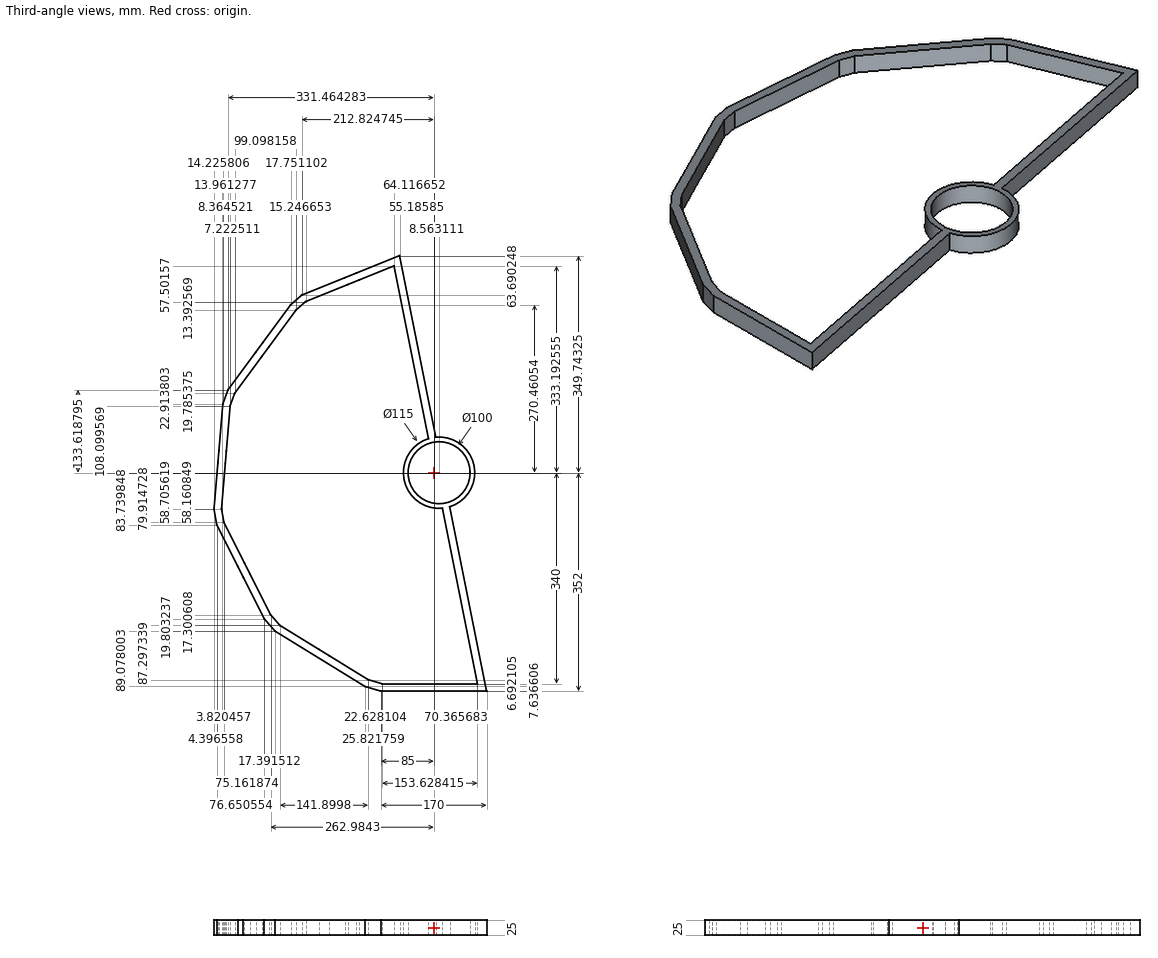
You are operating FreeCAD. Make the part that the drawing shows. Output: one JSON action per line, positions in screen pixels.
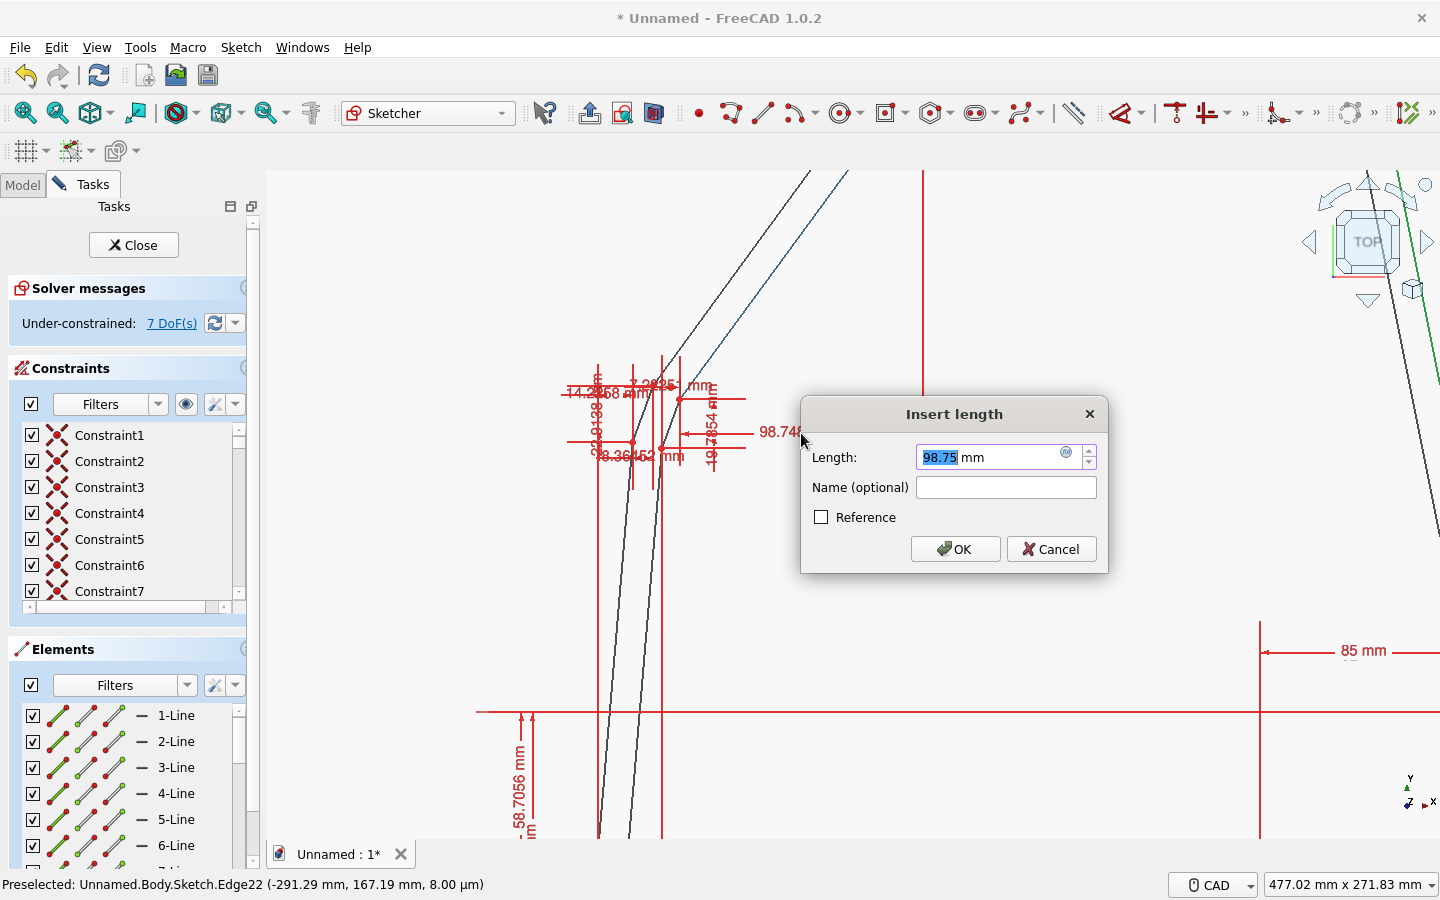
{"action": "type", "text": "99.098158"}
{"action": "key", "text": "Return"}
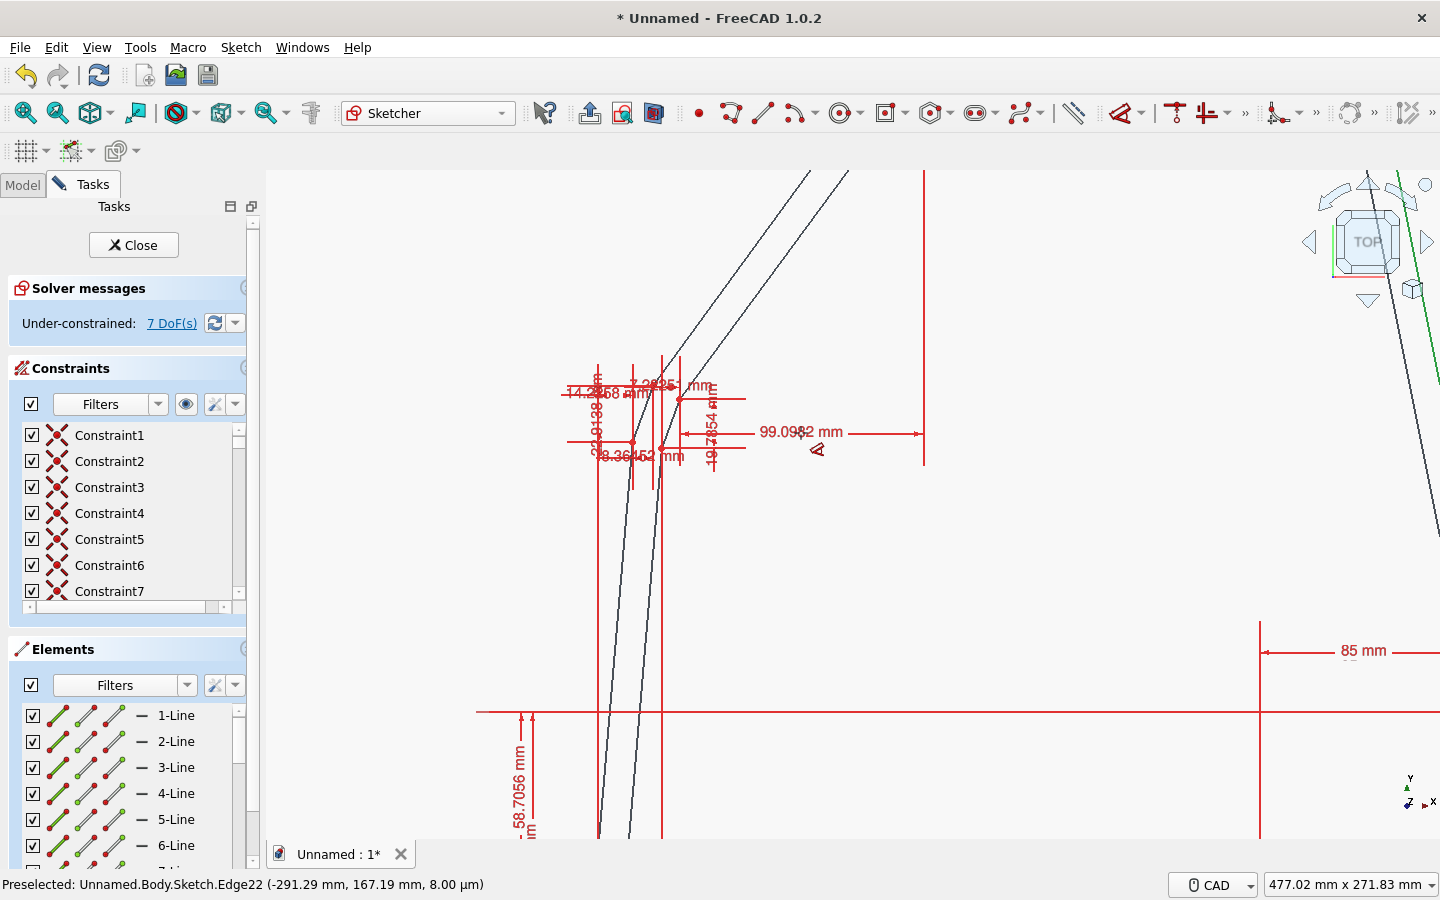
{"action": "scroll", "coordinate": [669, 436], "scroll_direction": "down", "scroll_amount": 7}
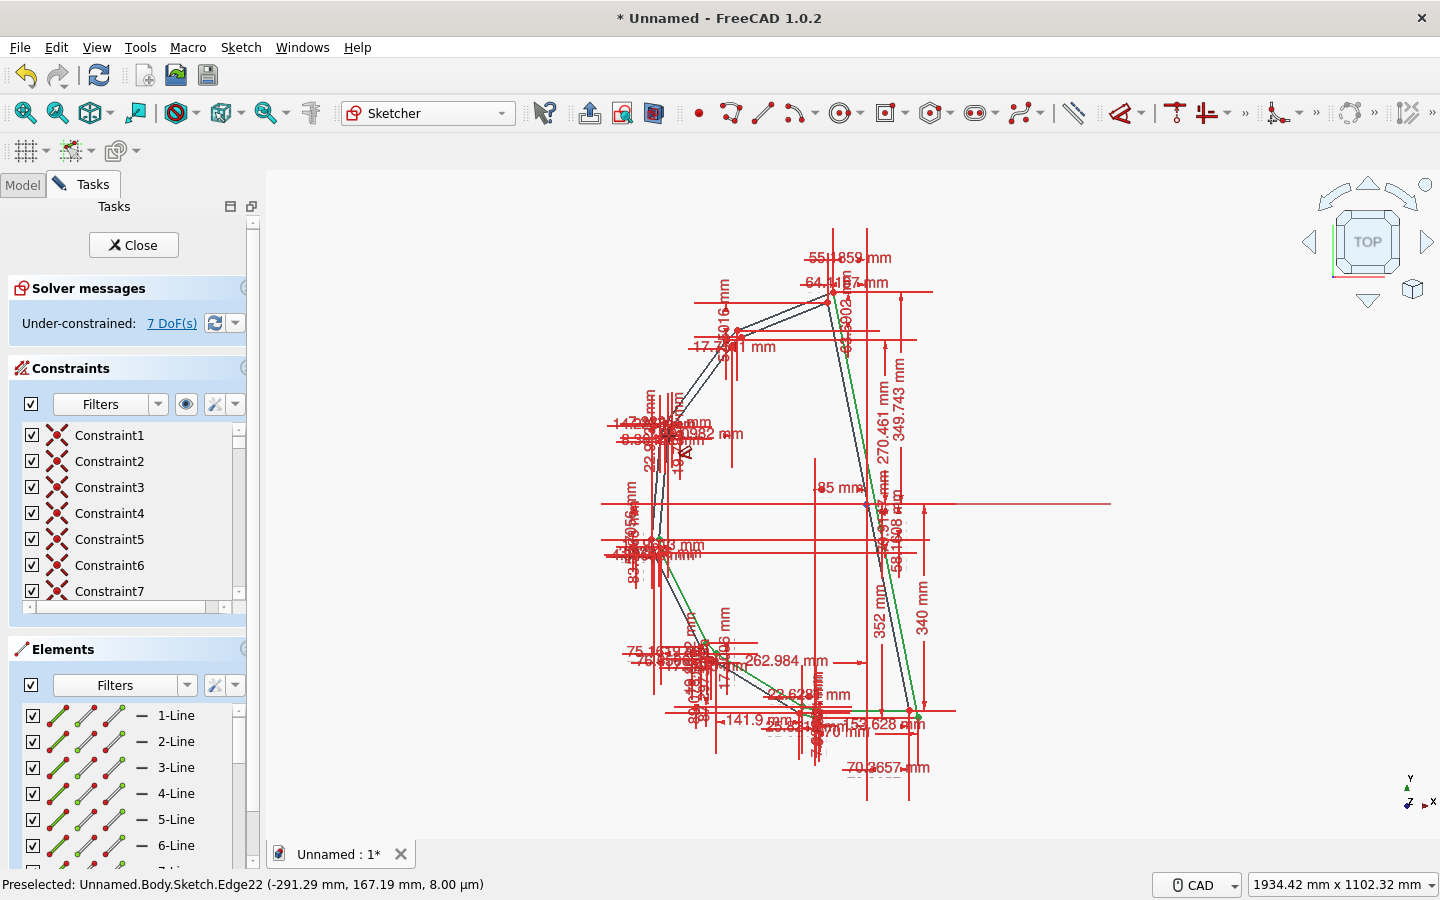
{"action": "scroll", "coordinate": [735, 343], "scroll_direction": "up", "scroll_amount": 8}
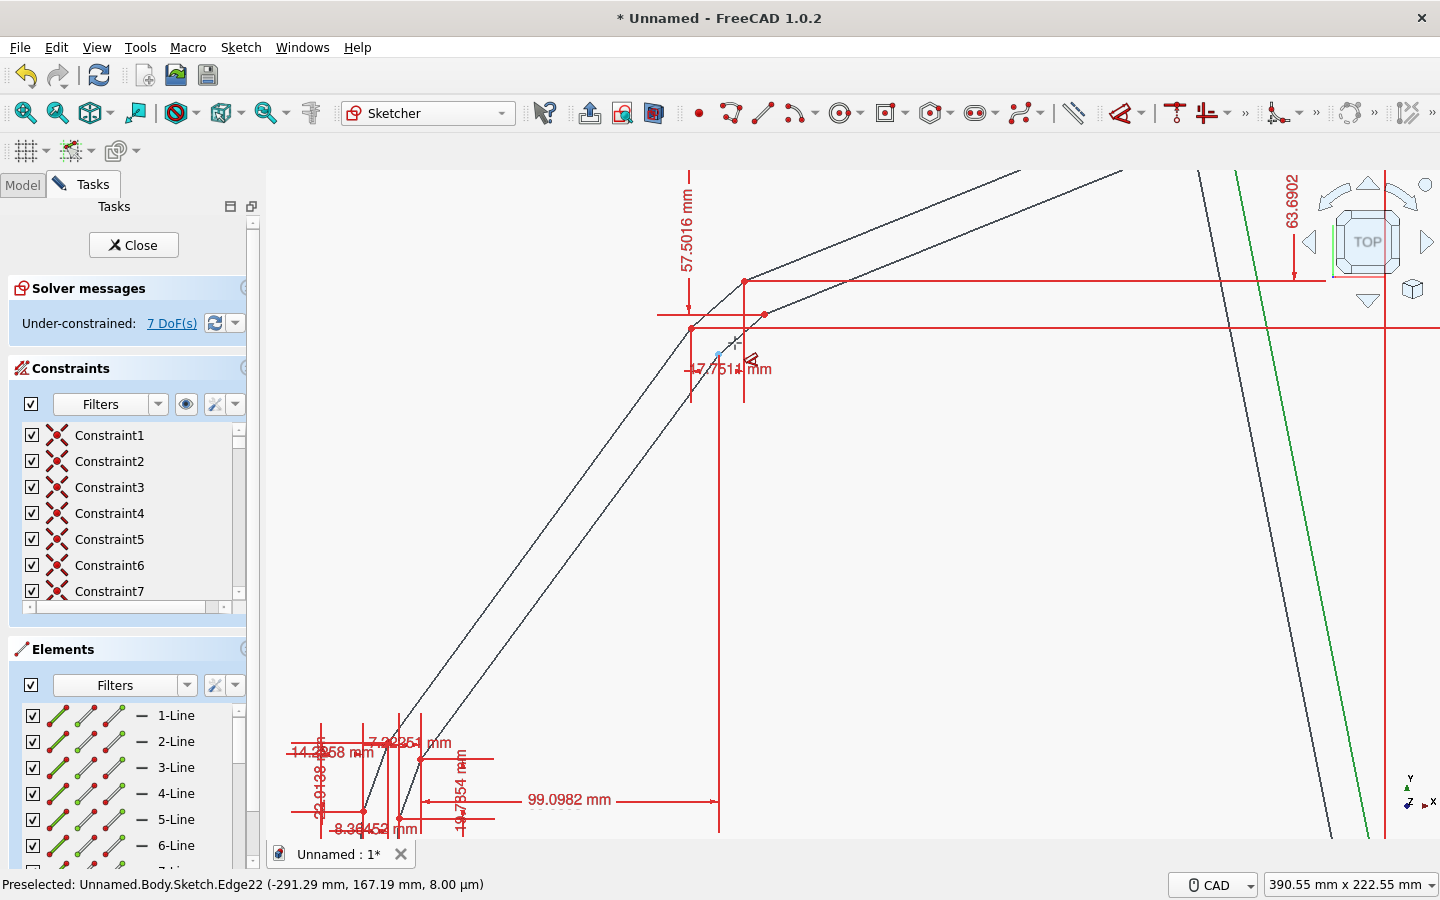
{"action": "left_click", "coordinate": [733, 343]}
{"action": "left_click", "coordinate": [742, 257]}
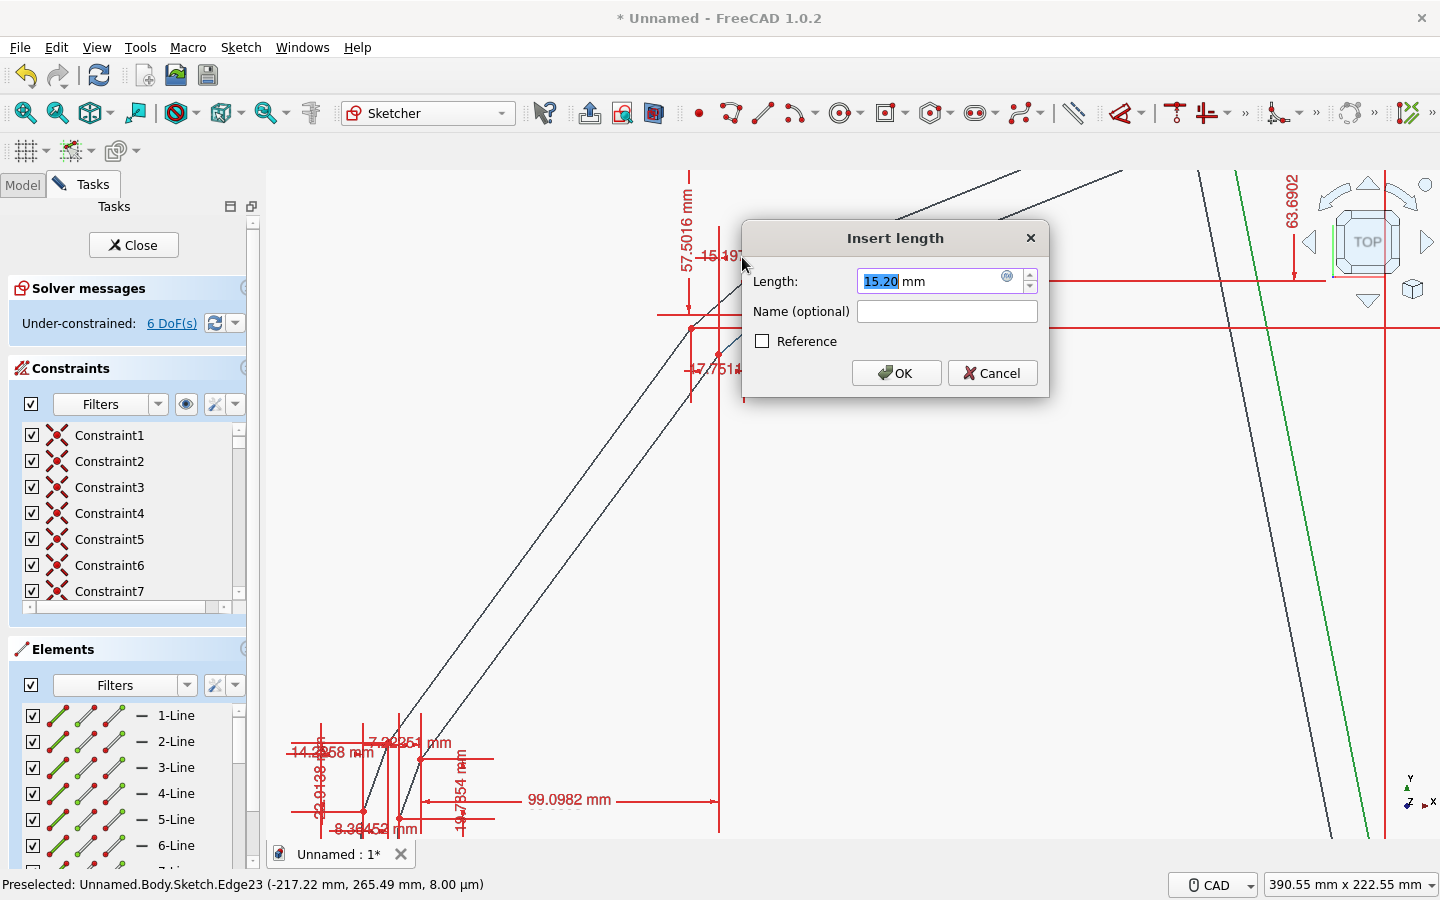
{"action": "type", "text": "15.246653"}
{"action": "key", "text": "Return"}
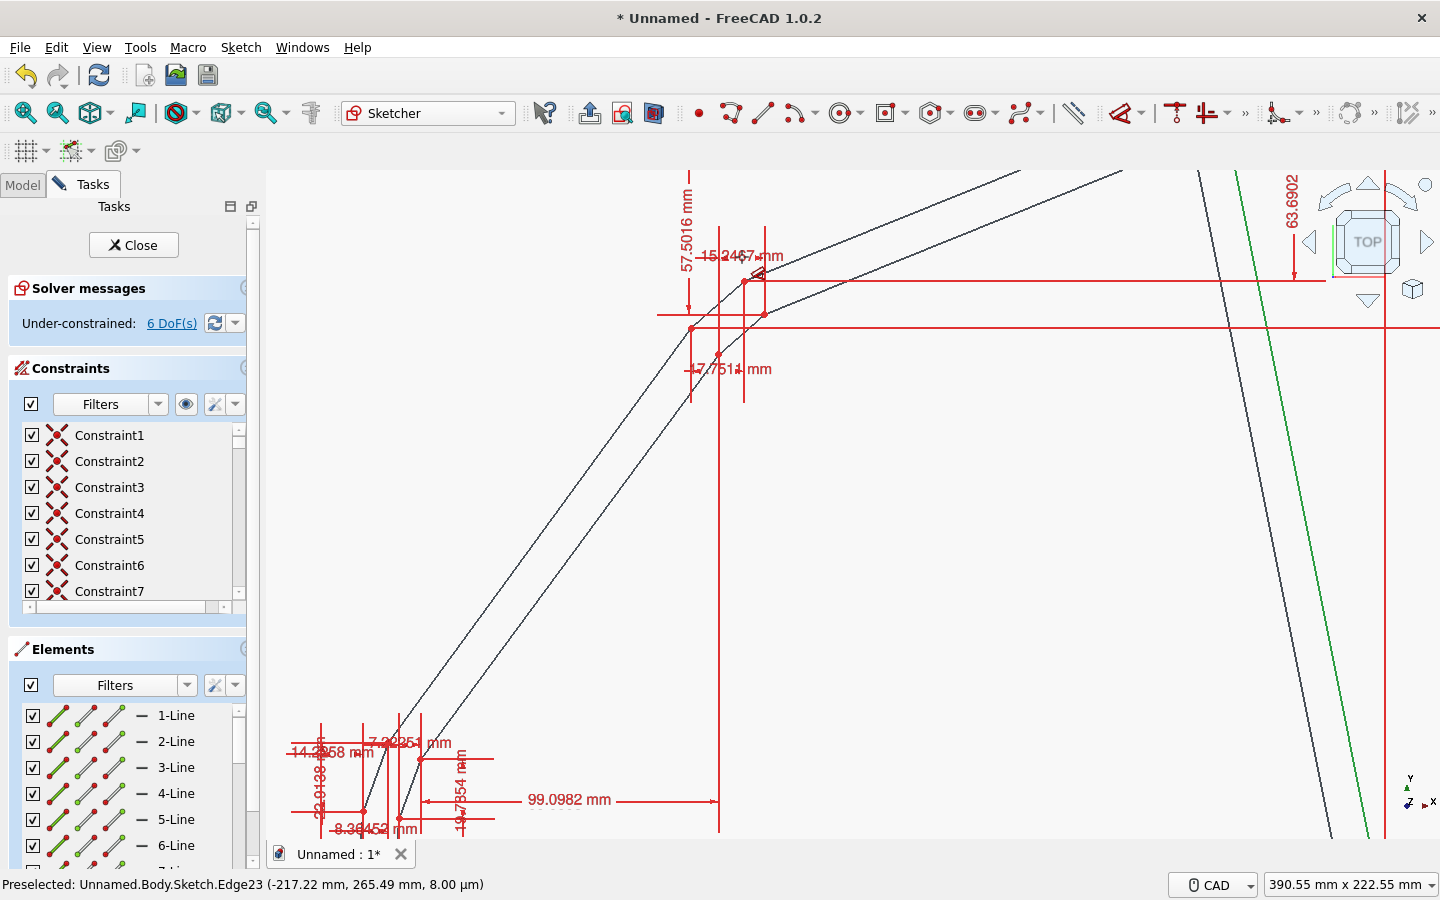
{"action": "left_click", "coordinate": [733, 343]}
{"action": "left_click", "coordinate": [799, 335]}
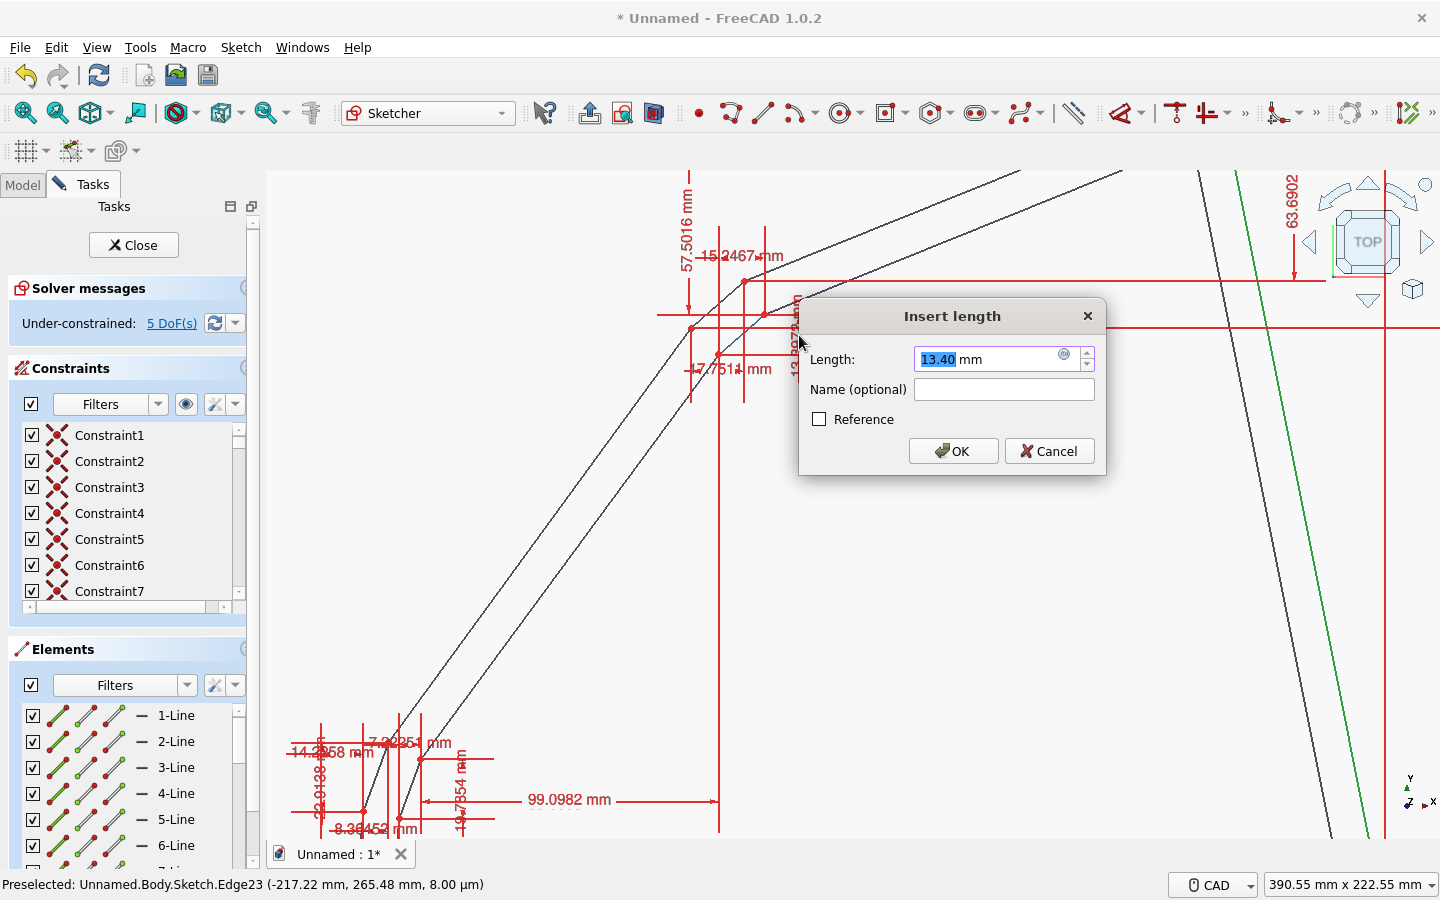
{"action": "type", "text": "13.392569"}
{"action": "key", "text": "Return"}